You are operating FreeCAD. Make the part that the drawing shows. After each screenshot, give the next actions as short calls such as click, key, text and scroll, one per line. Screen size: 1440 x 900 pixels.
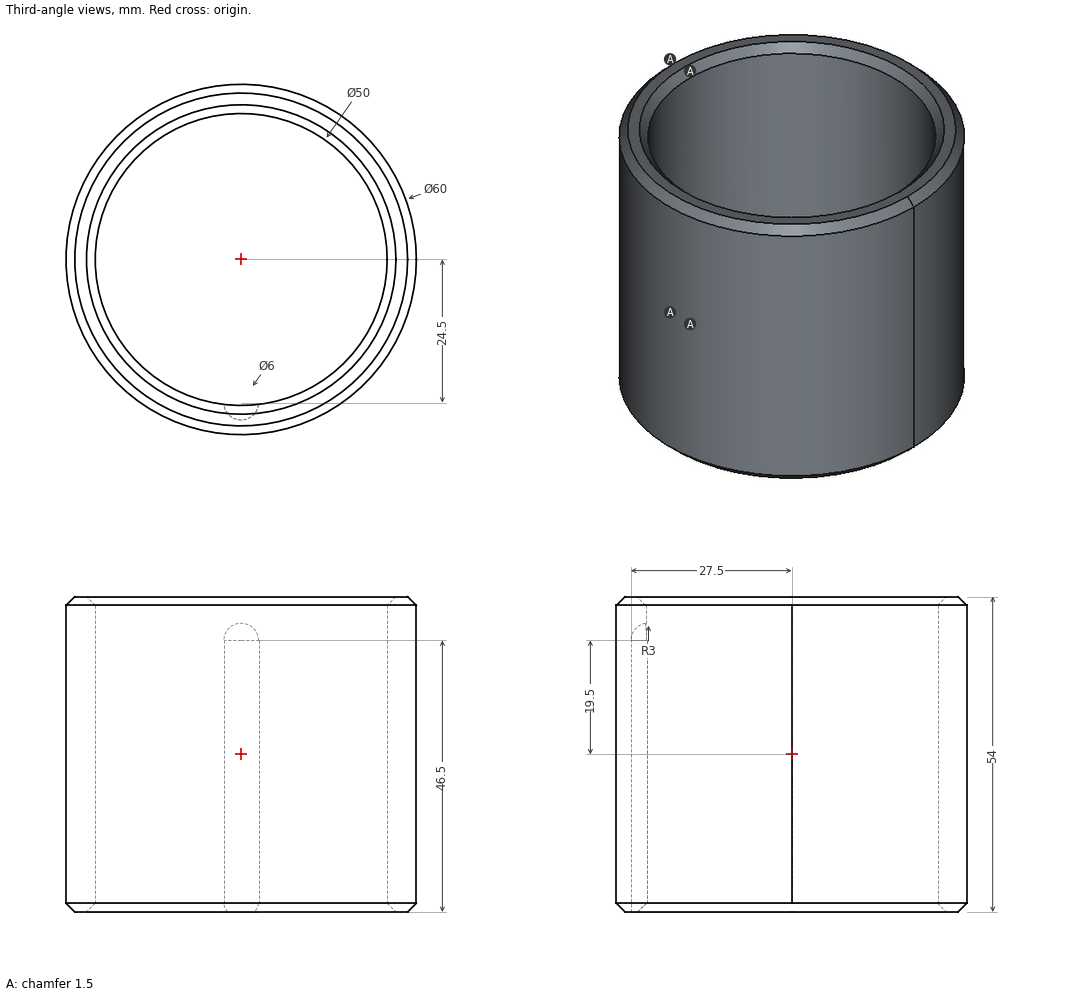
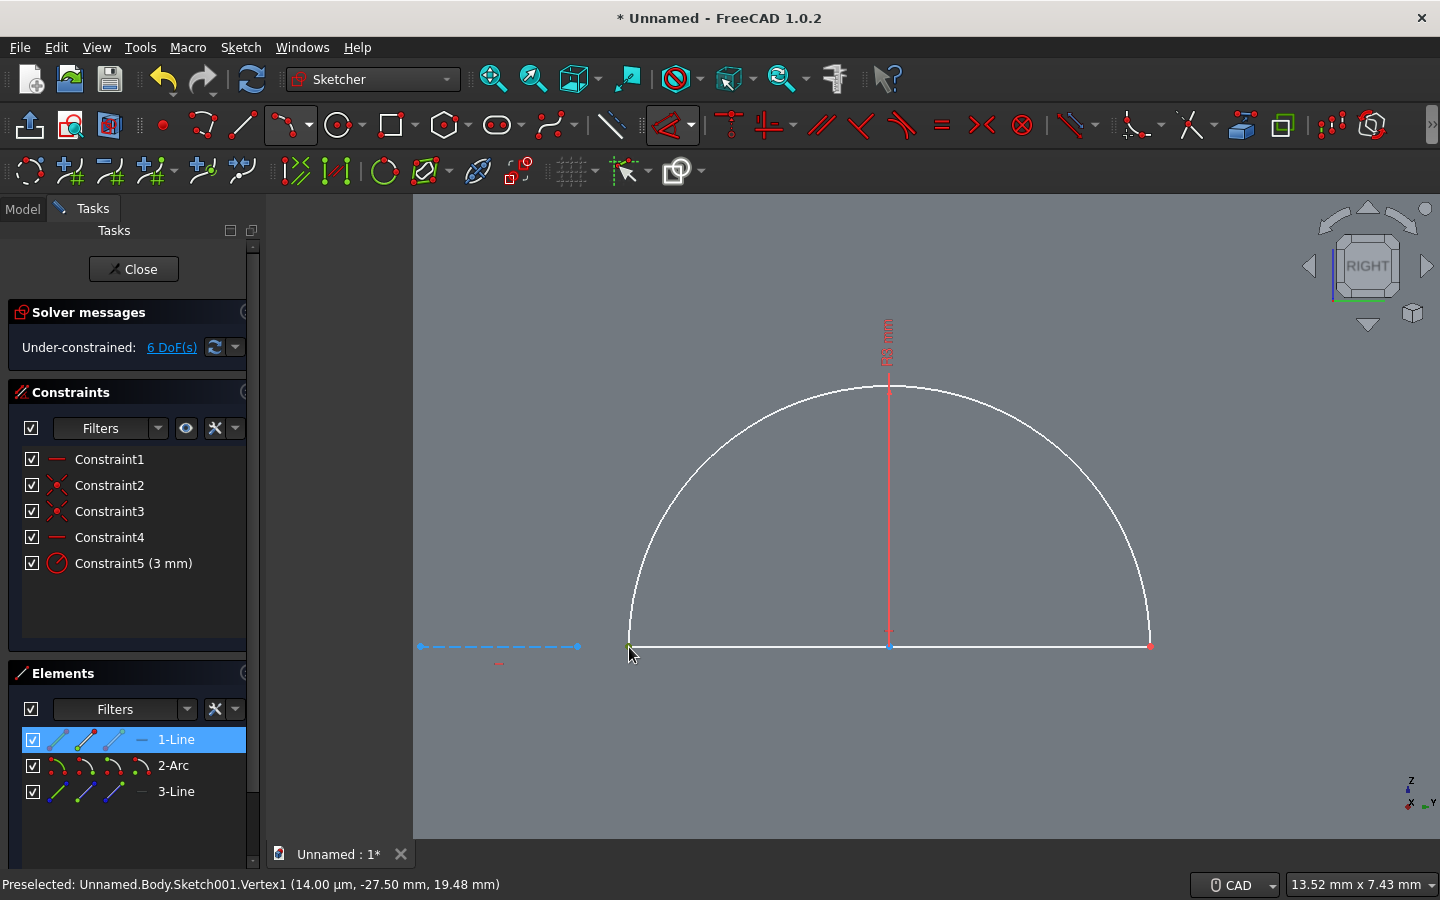
click(694, 126)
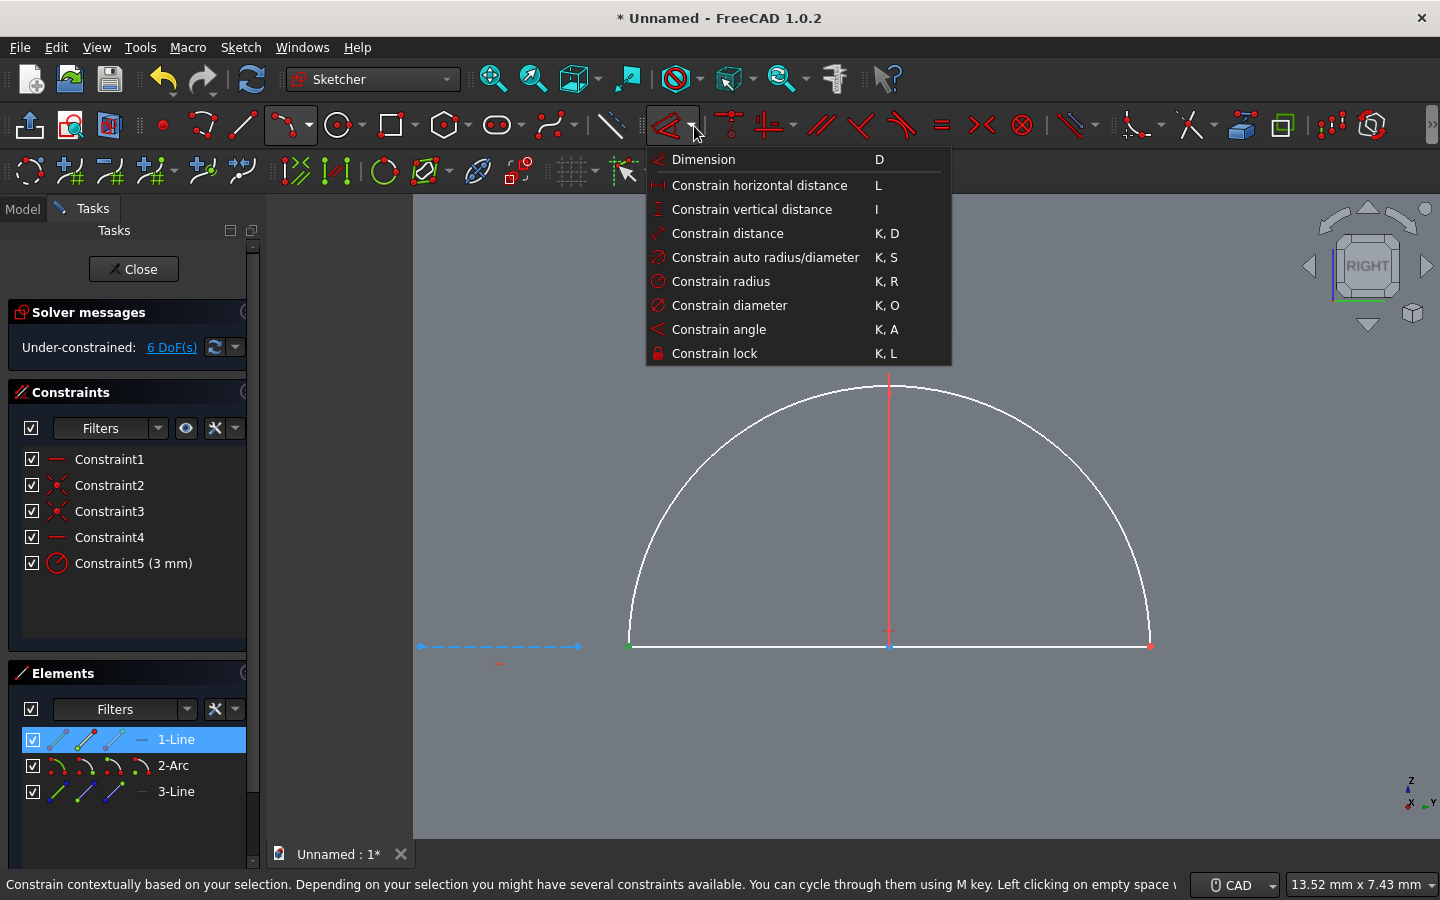
click(799, 185)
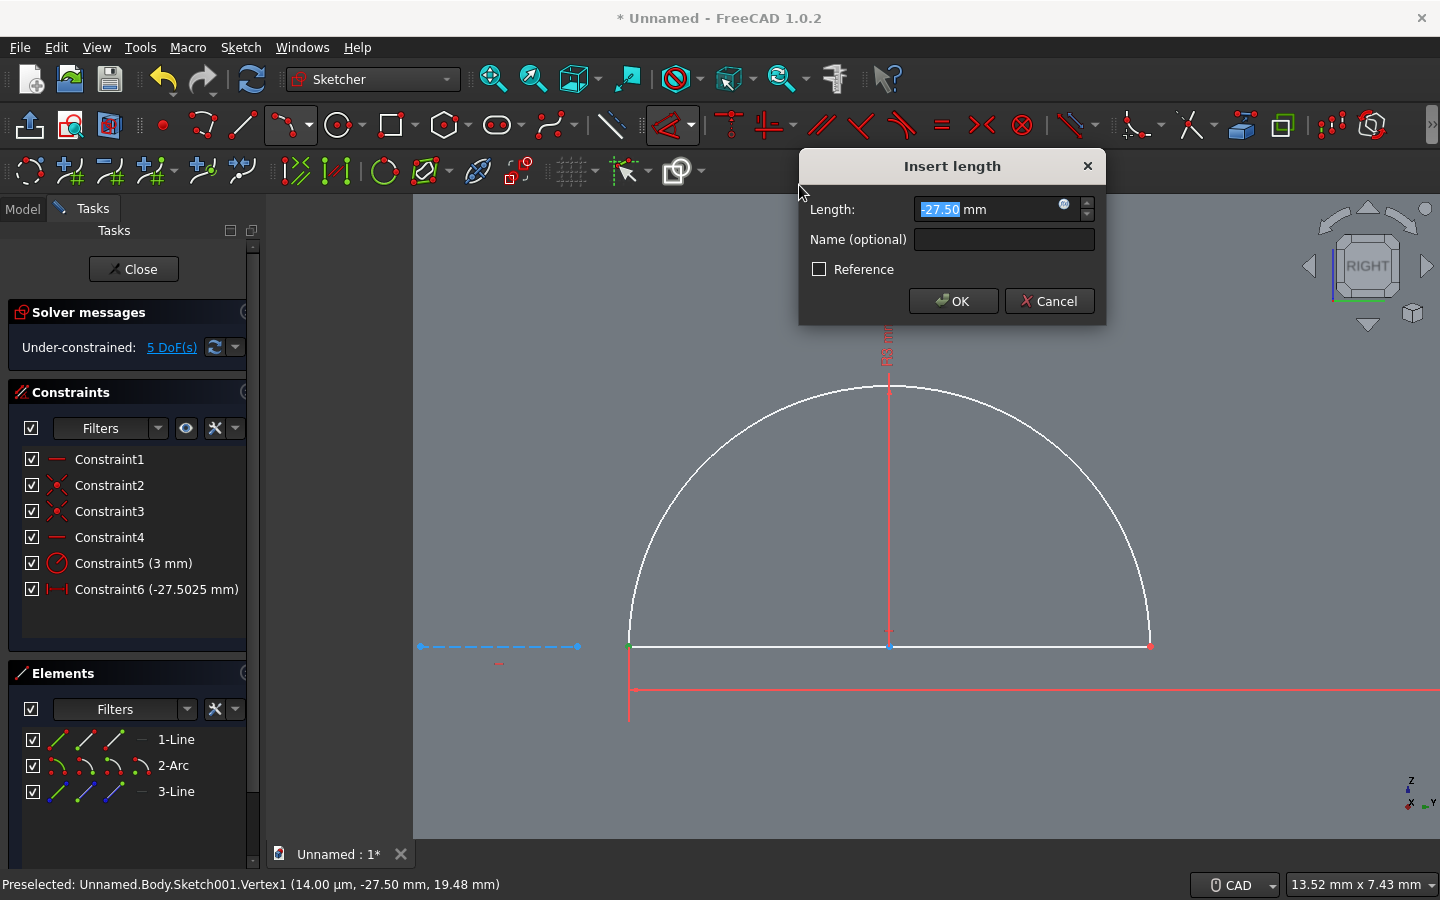
text(-27.5)
key(Return)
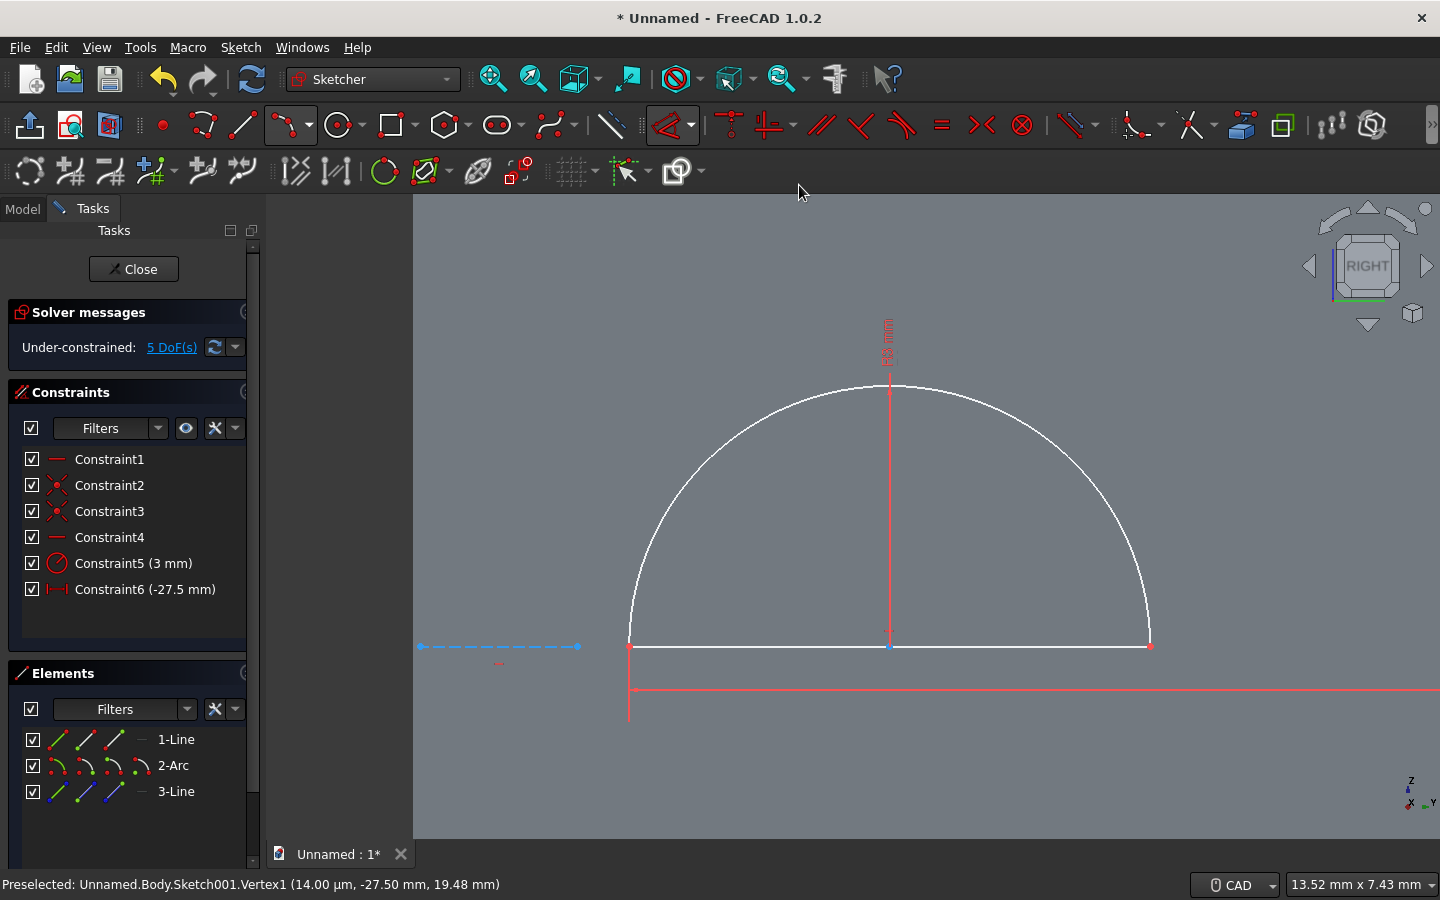
click(629, 647)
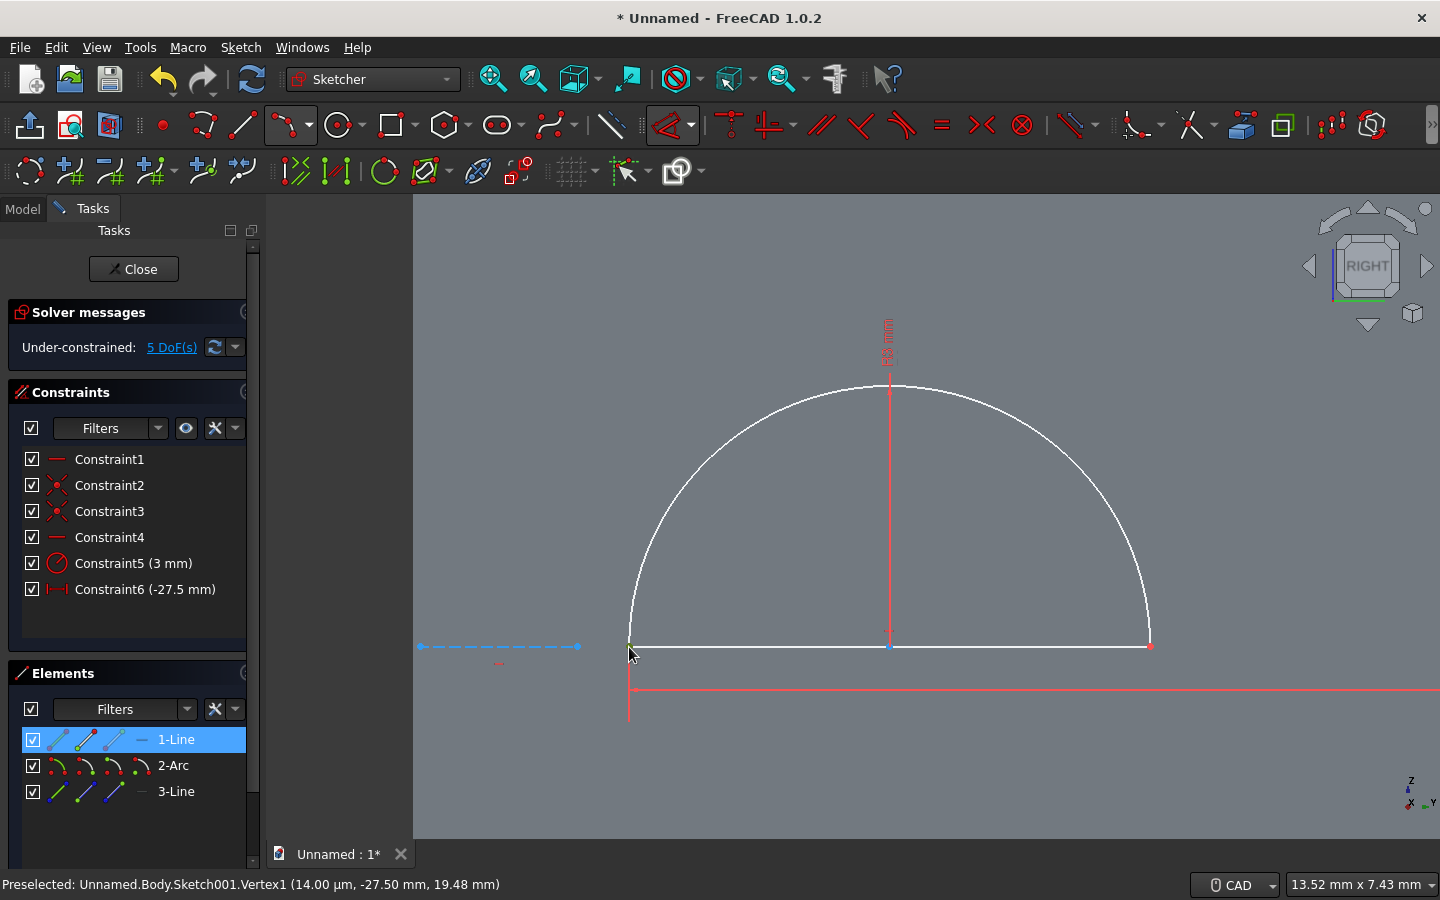
key(i)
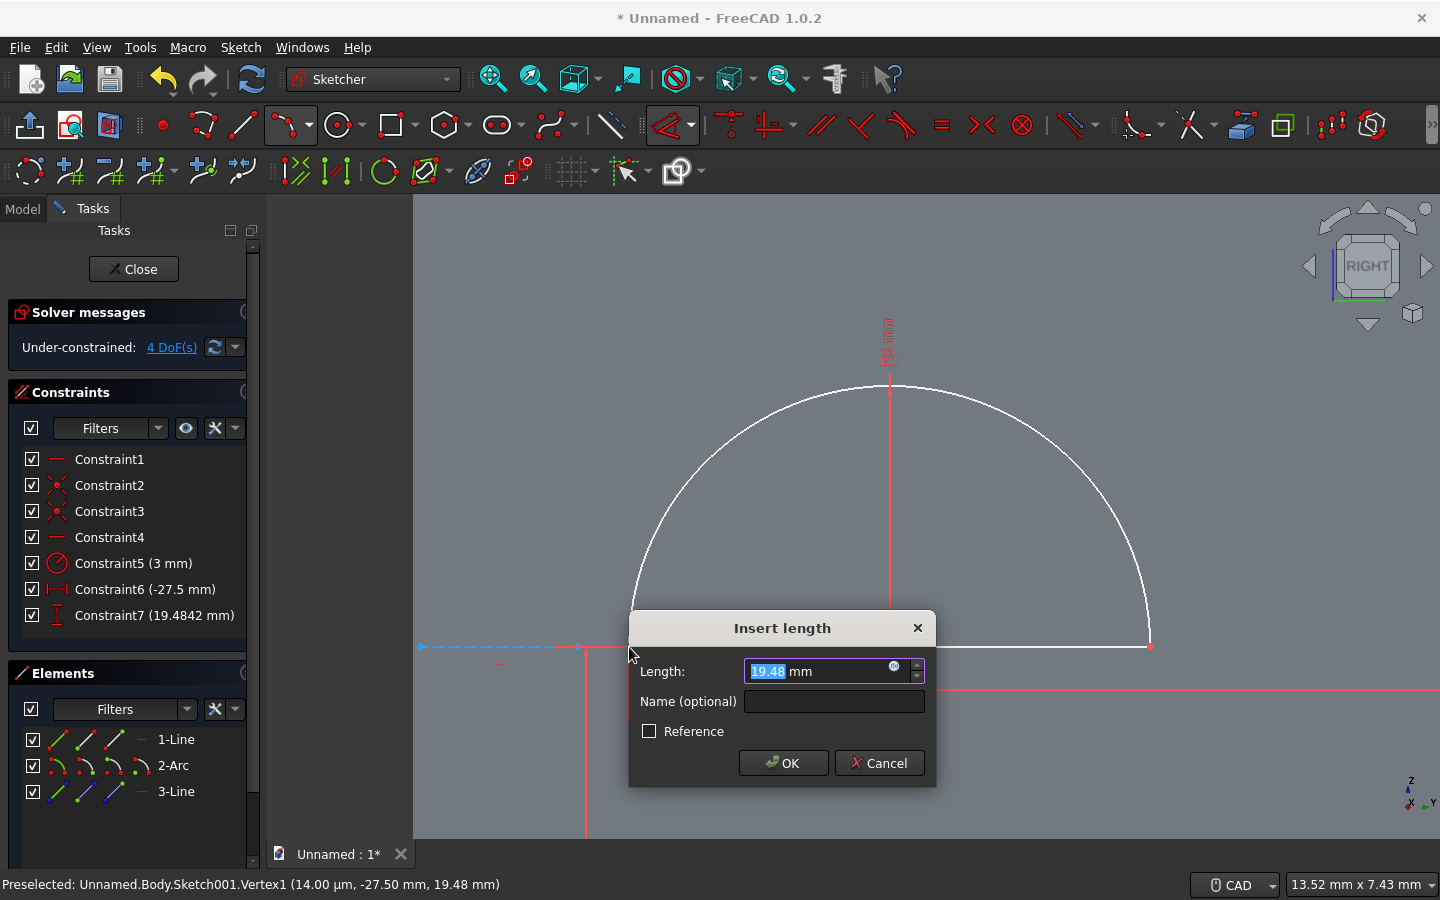
text(19.5)
key(Return)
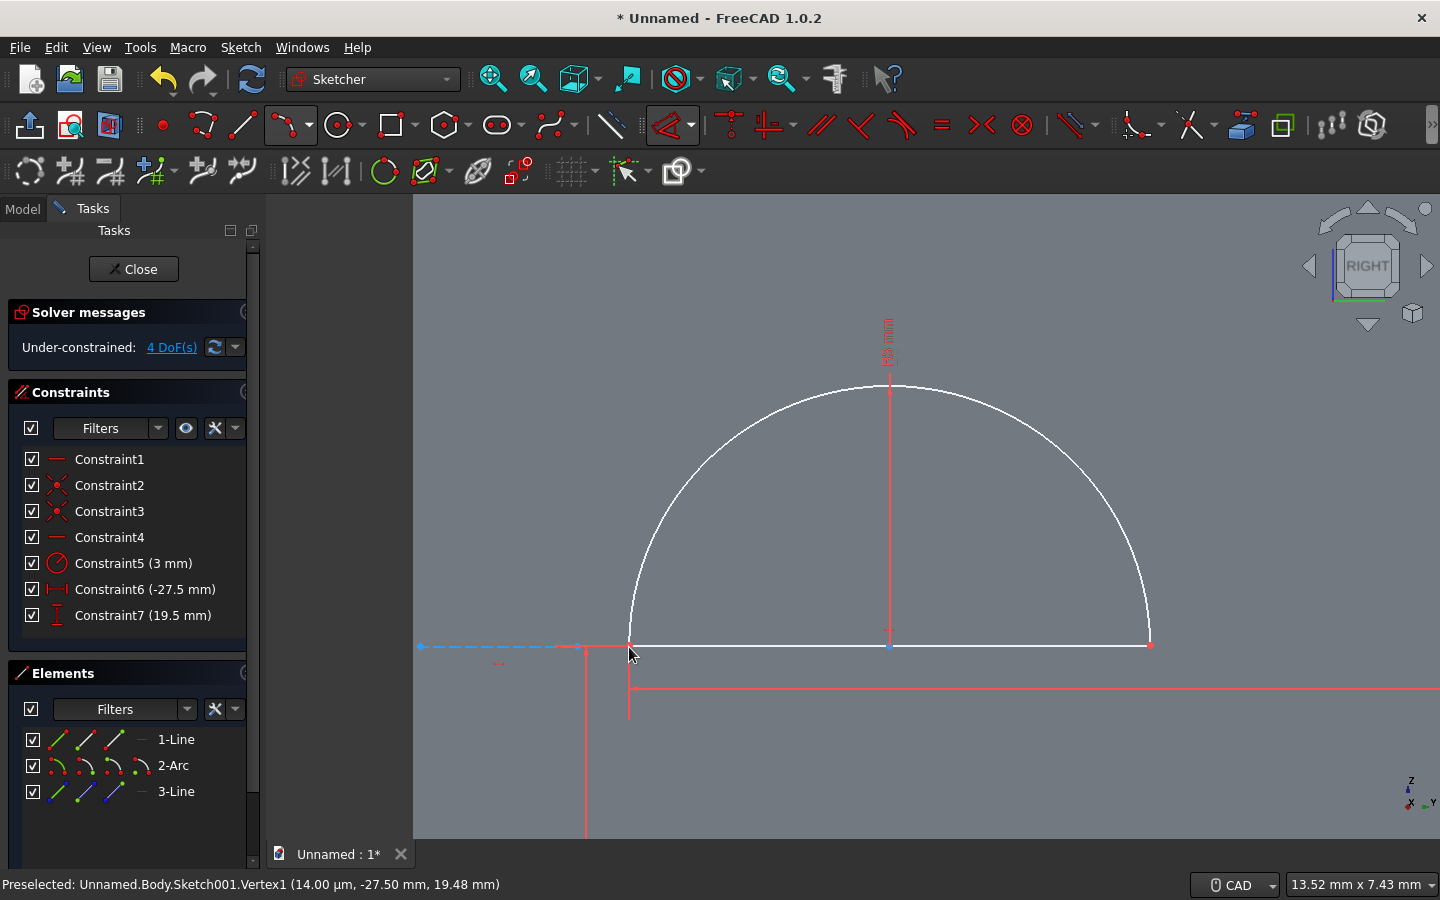
click(577, 647)